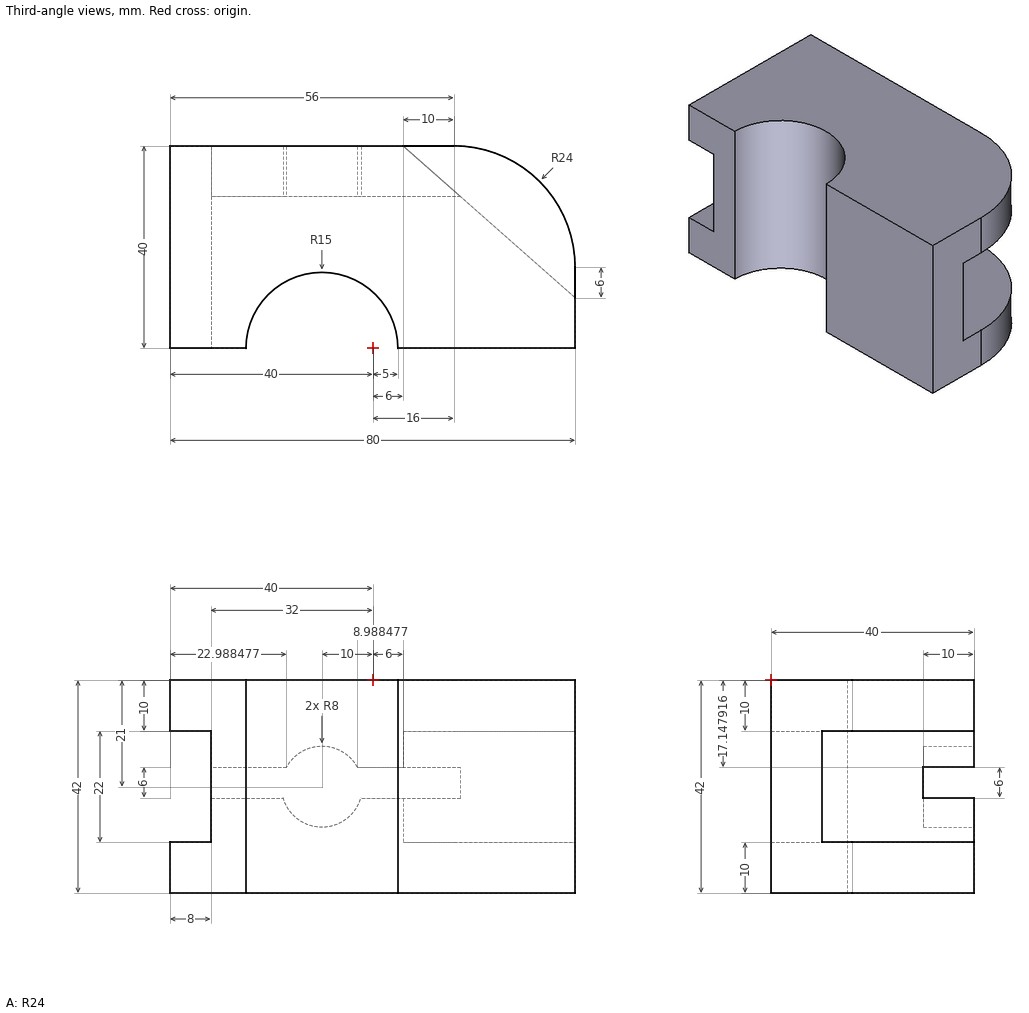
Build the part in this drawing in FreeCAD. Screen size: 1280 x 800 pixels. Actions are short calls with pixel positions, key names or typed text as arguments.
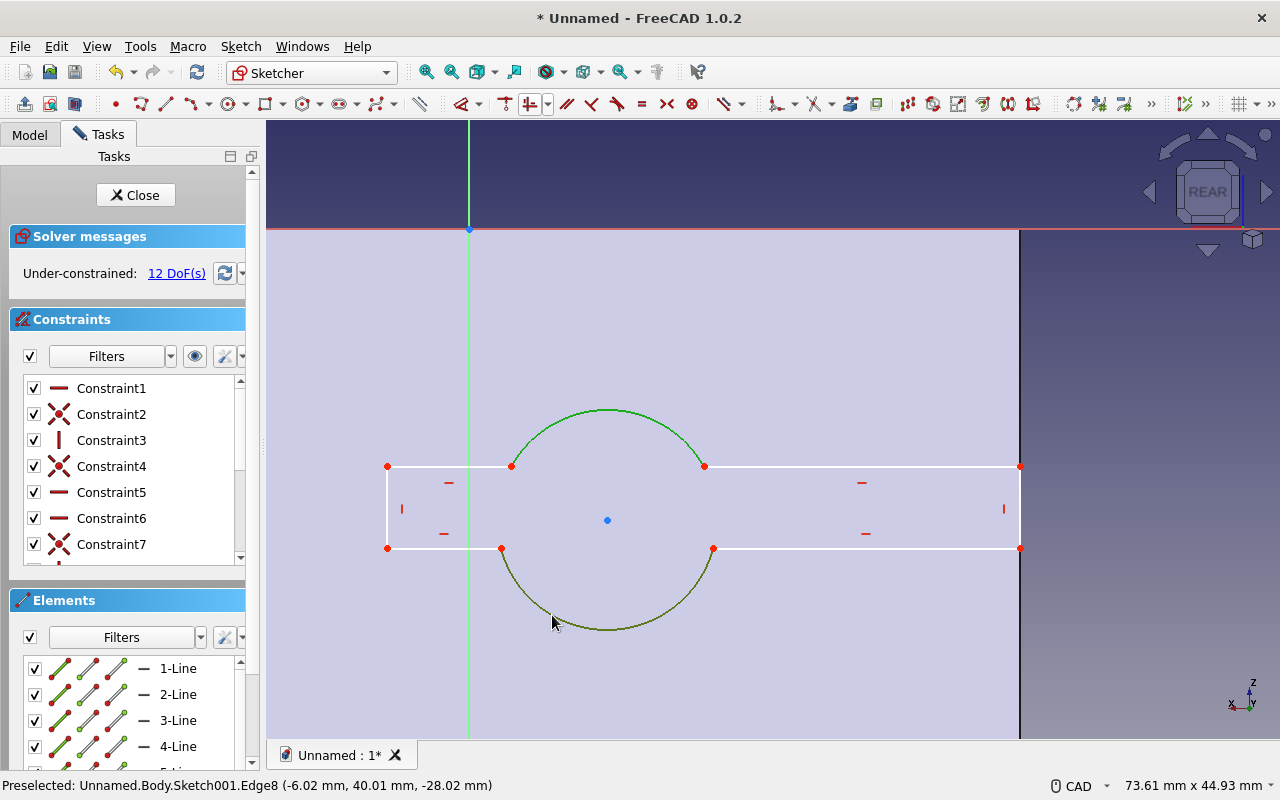
key(c)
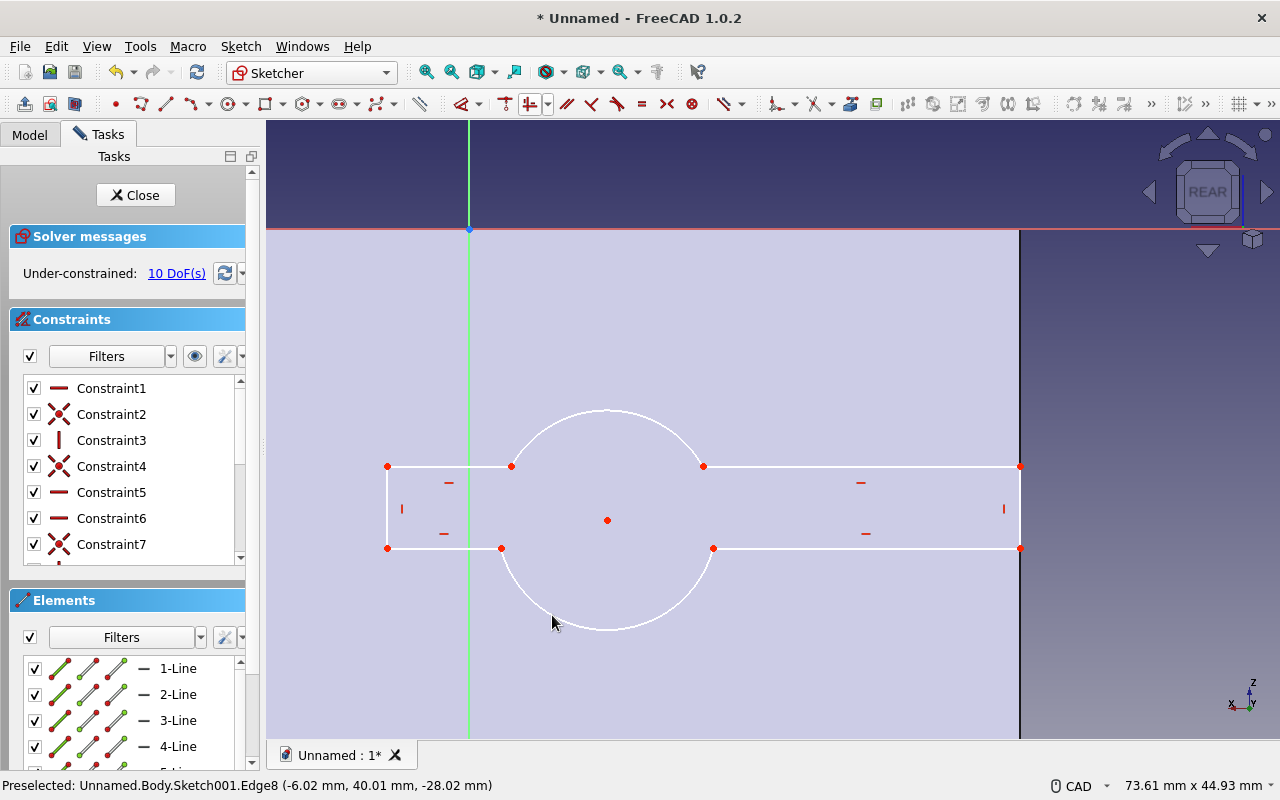
click(652, 420)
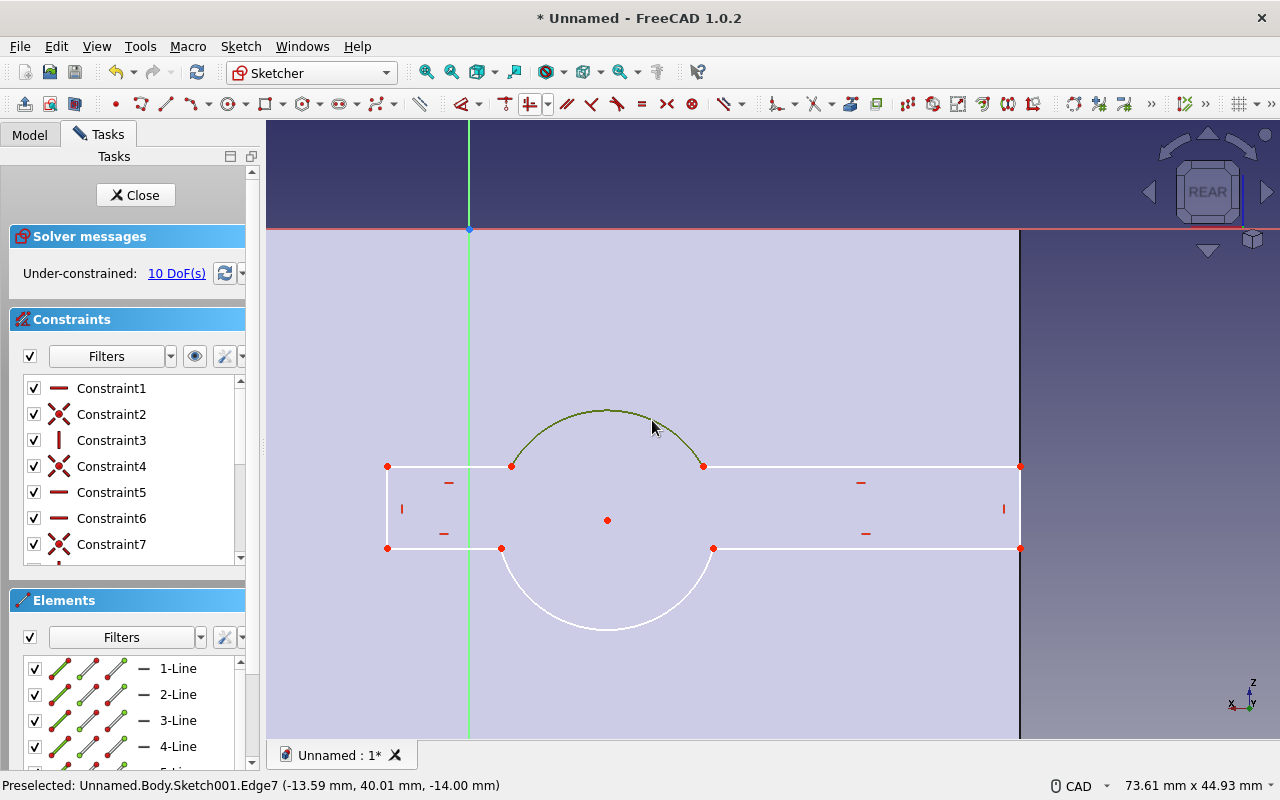
click(552, 615)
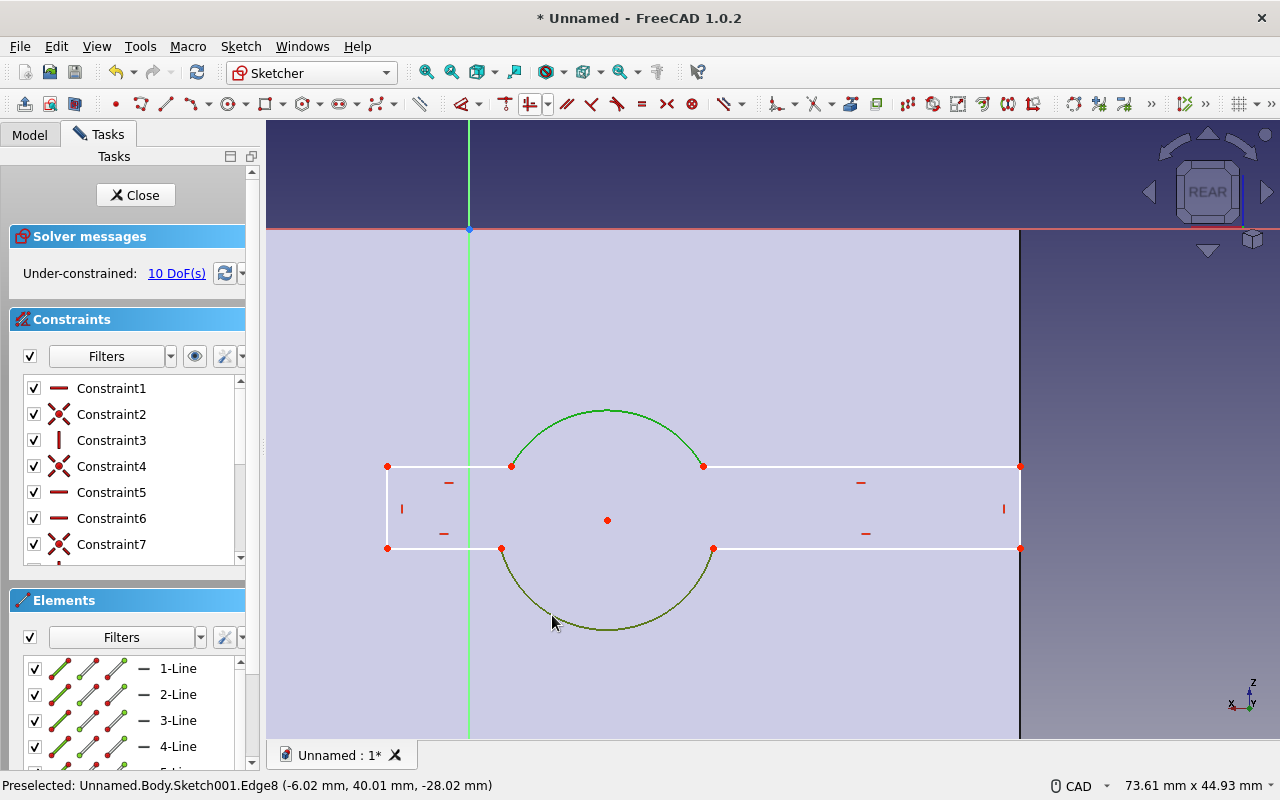
click(642, 104)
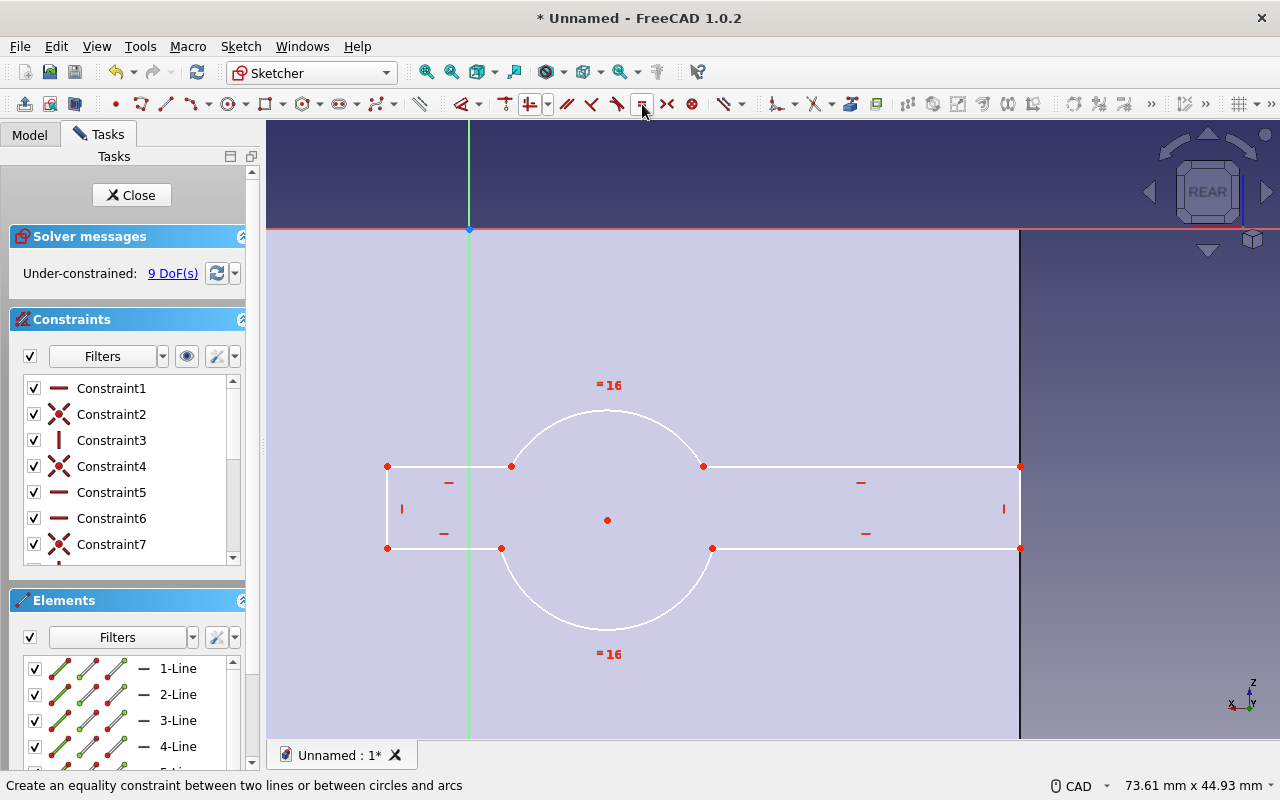
click(460, 104)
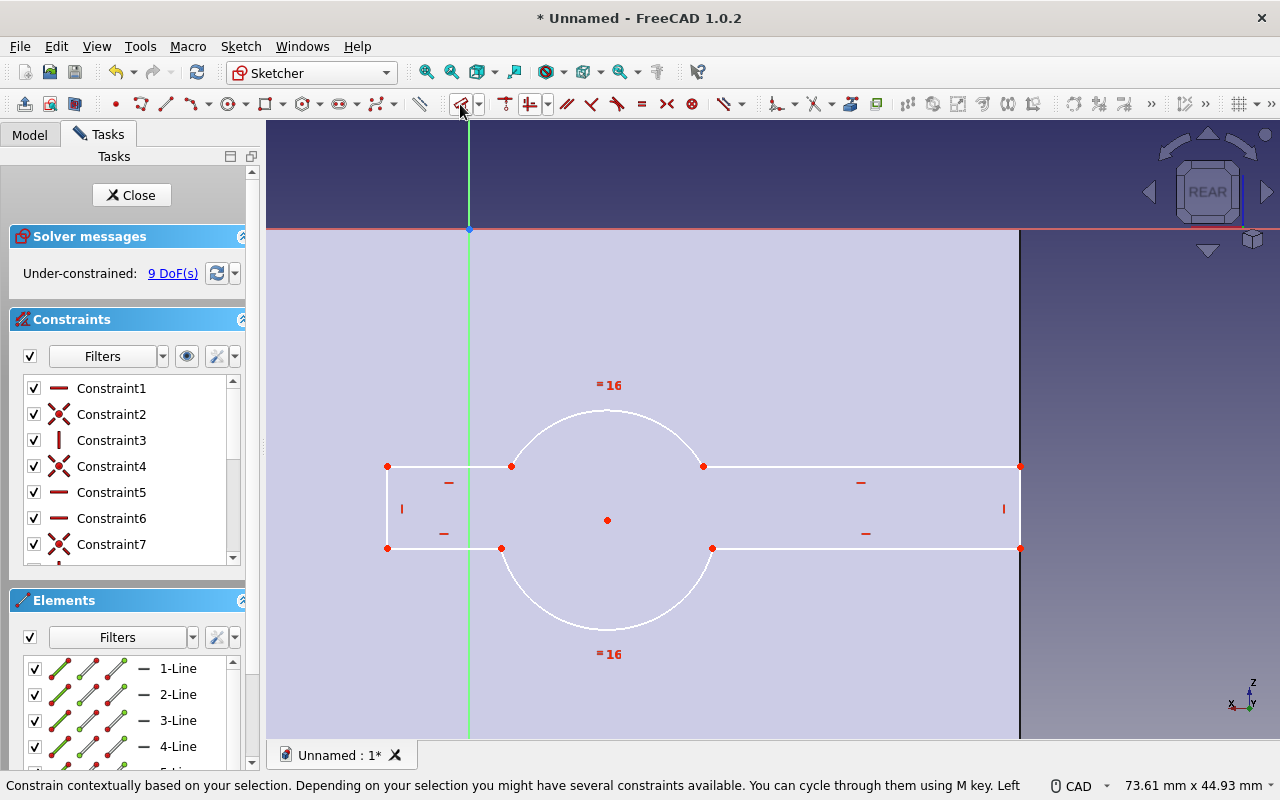
click(652, 420)
click(665, 391)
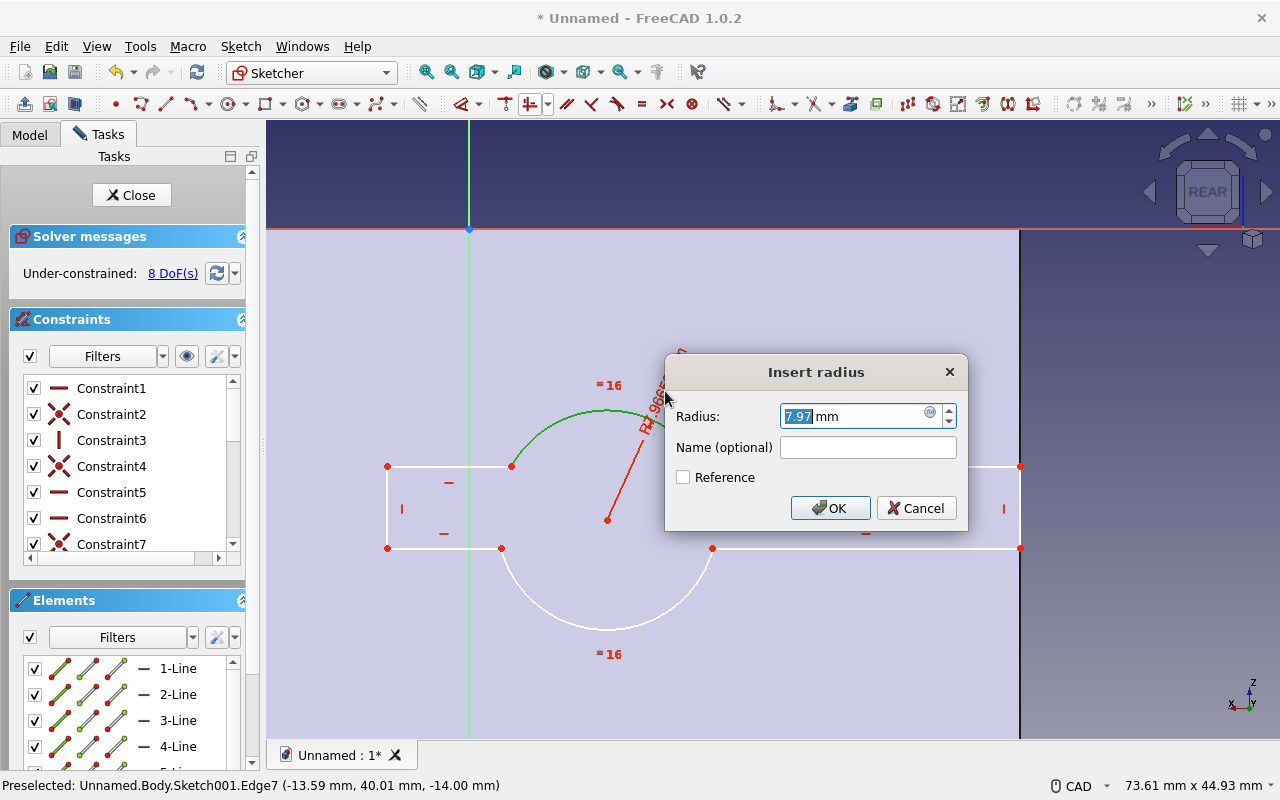
text(8)
key(Return)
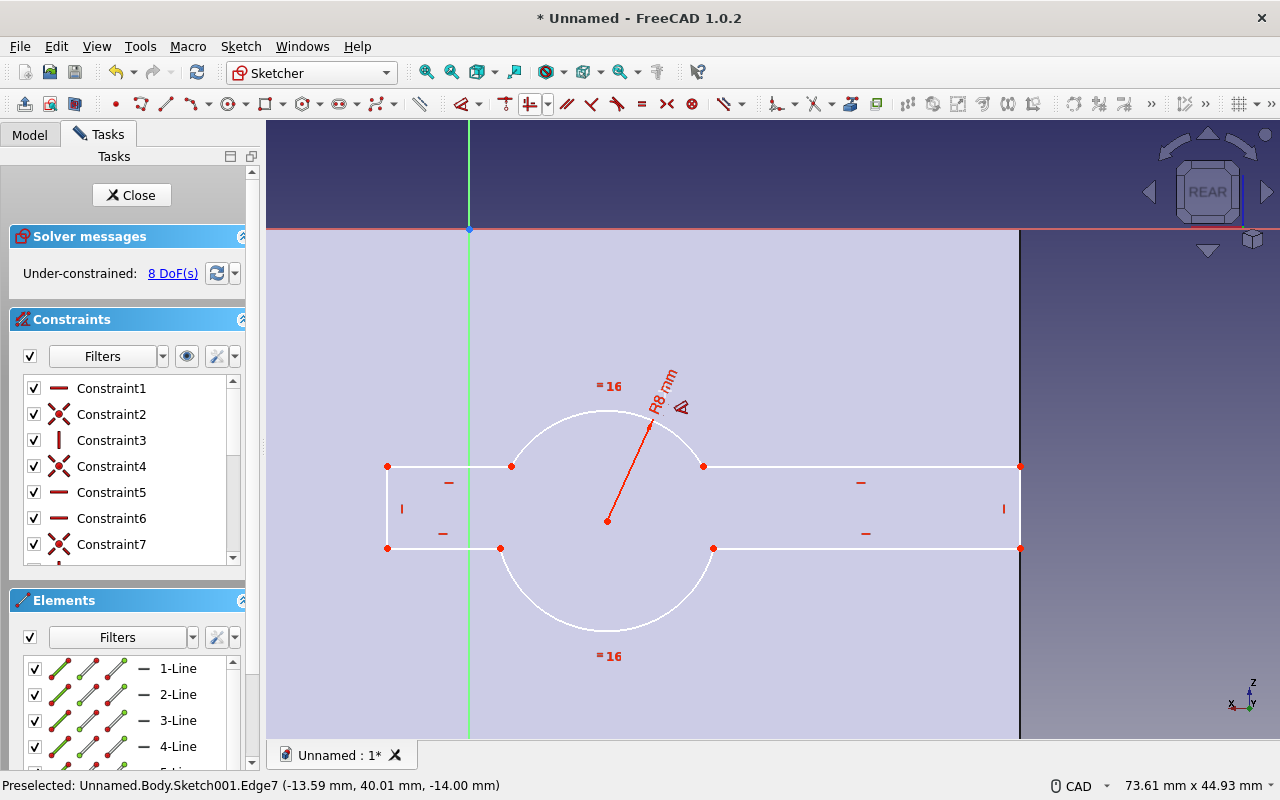
click(1020, 524)
click(1054, 508)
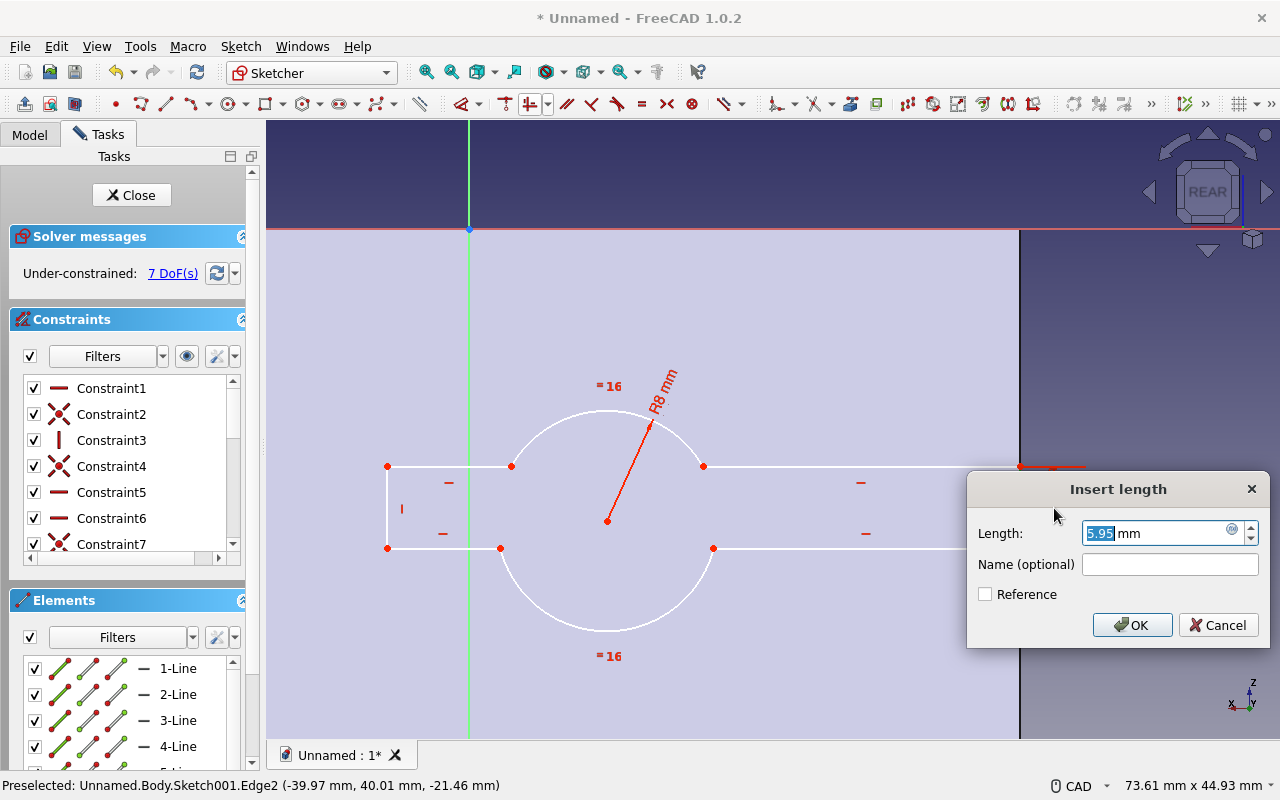
text(6)
key(Return)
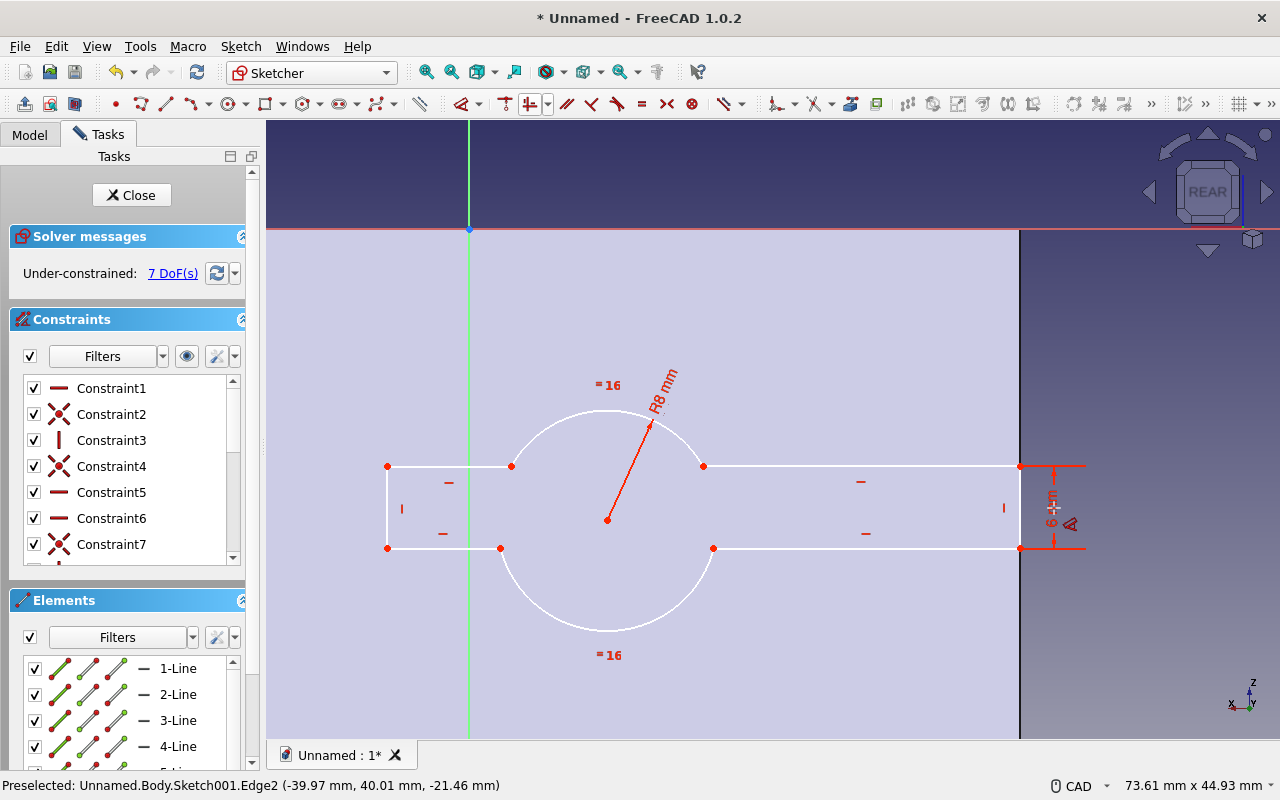
click(387, 492)
click(353, 508)